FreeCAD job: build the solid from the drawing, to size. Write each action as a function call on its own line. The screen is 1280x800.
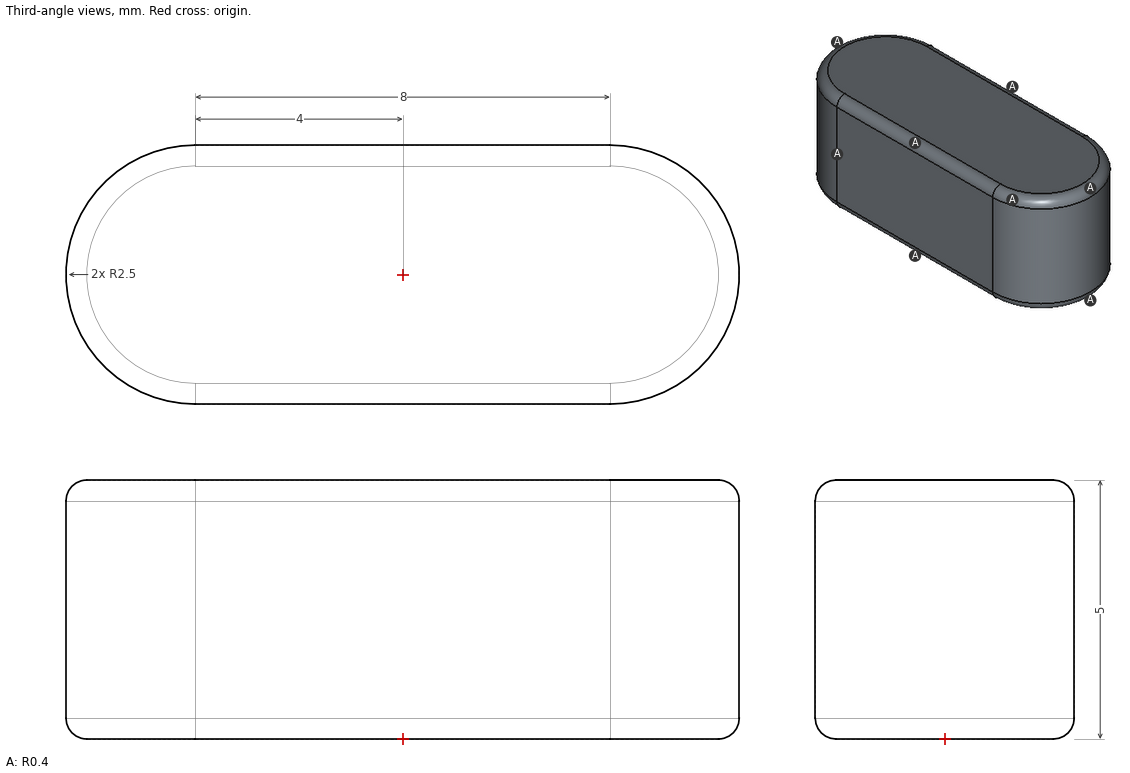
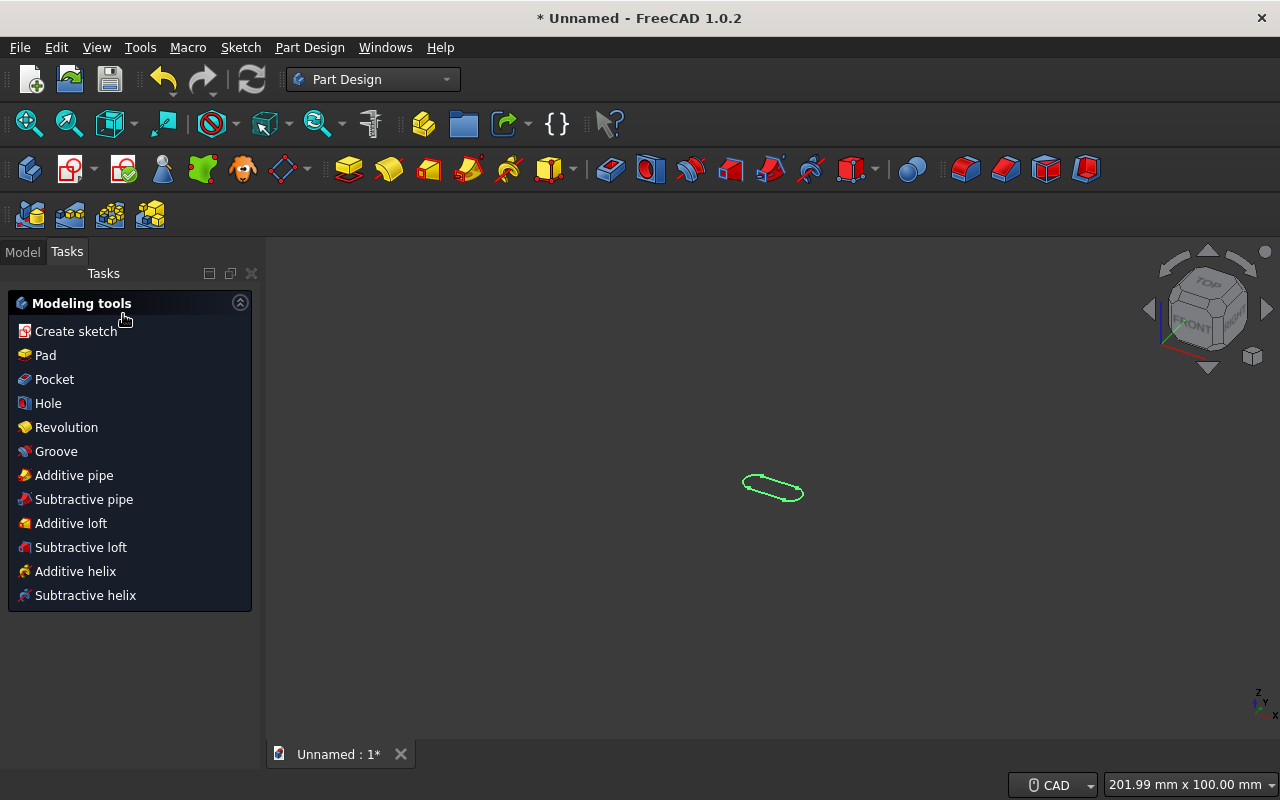
click(350, 170)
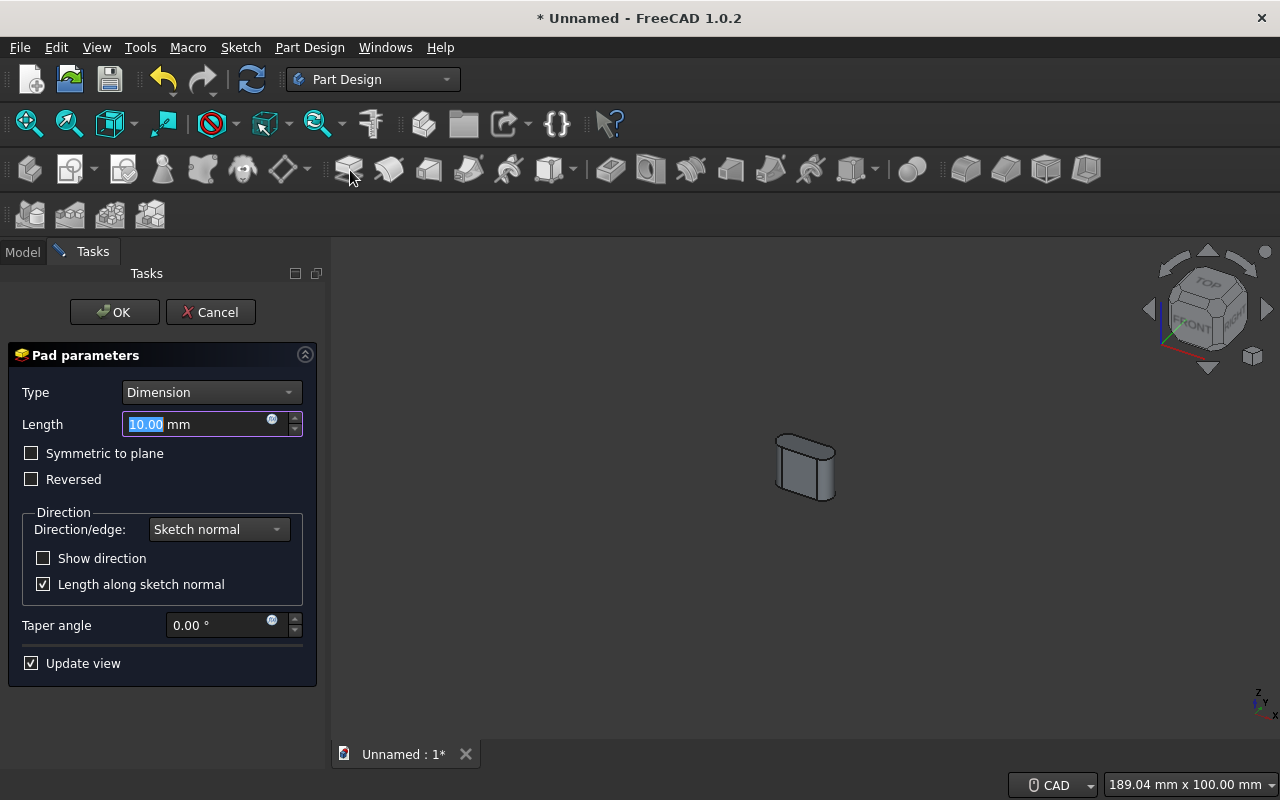
text(5)
key(Tab)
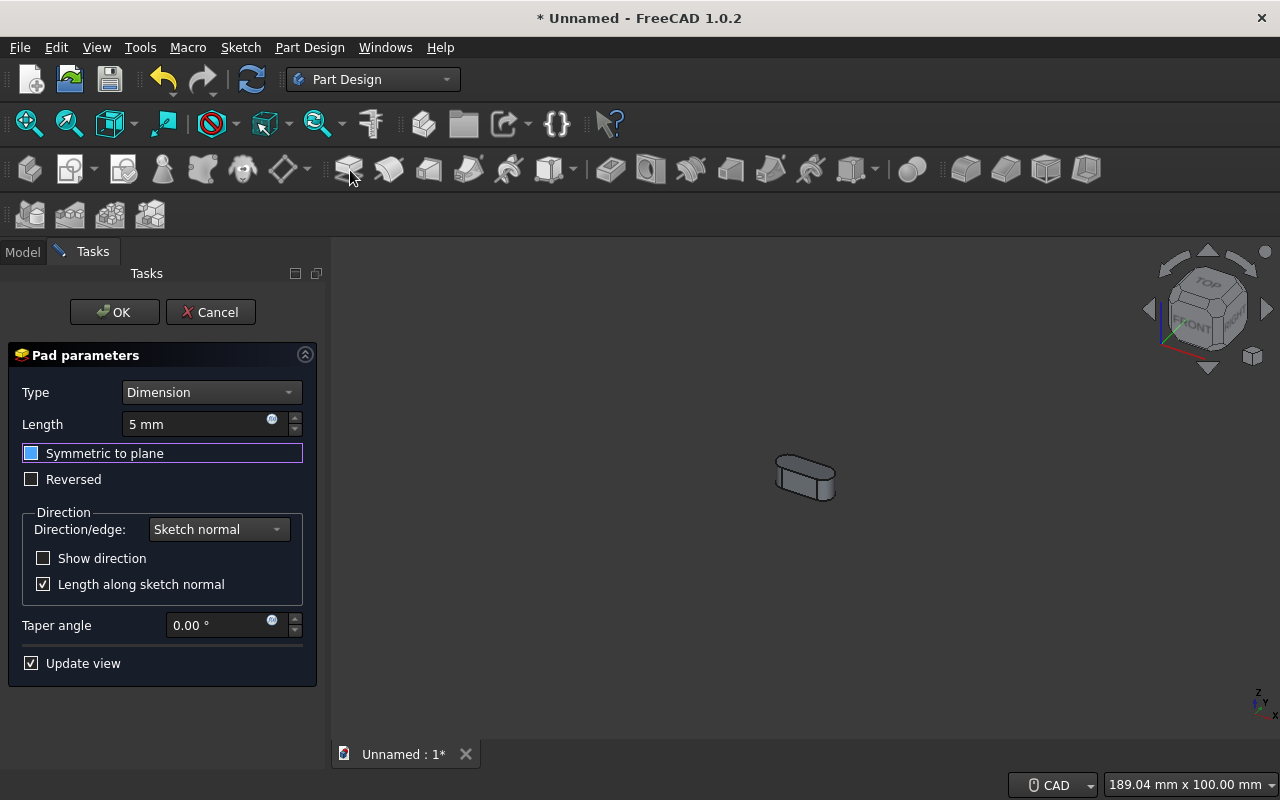
click(115, 312)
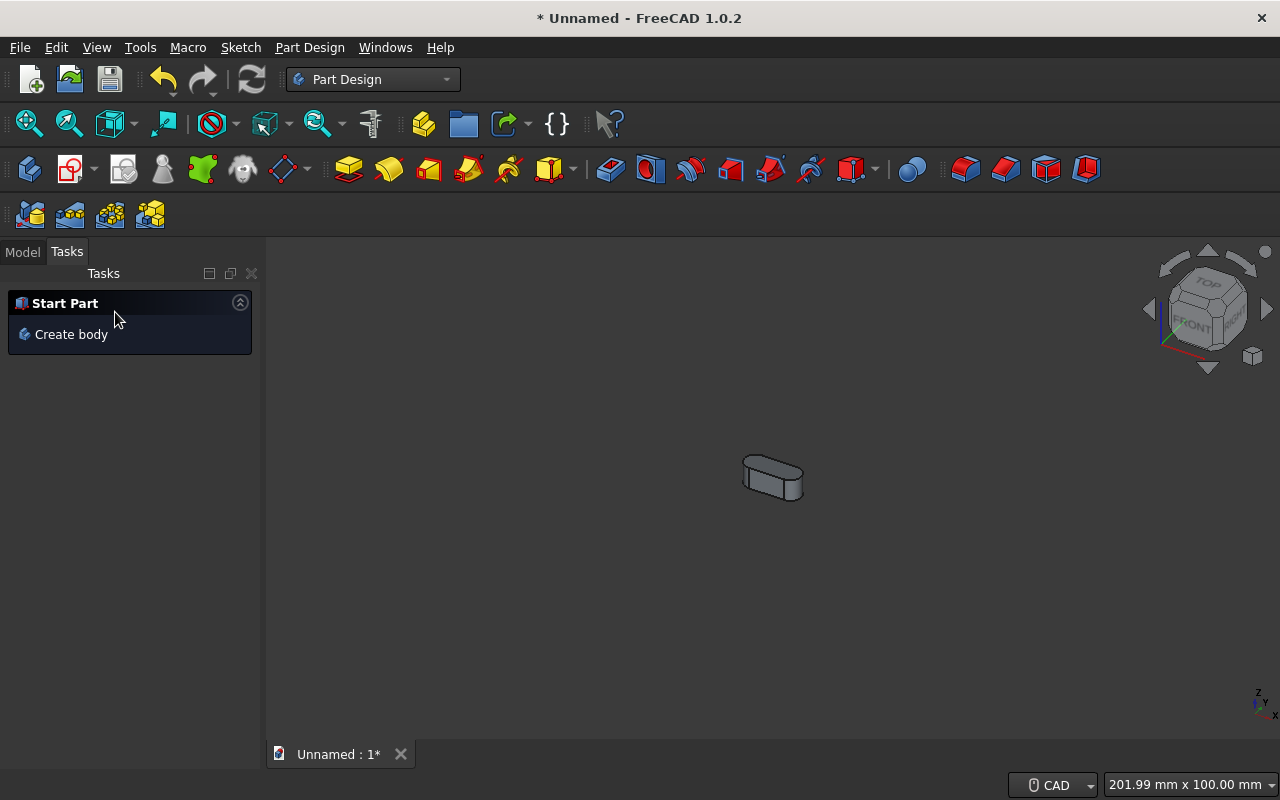
click(30, 124)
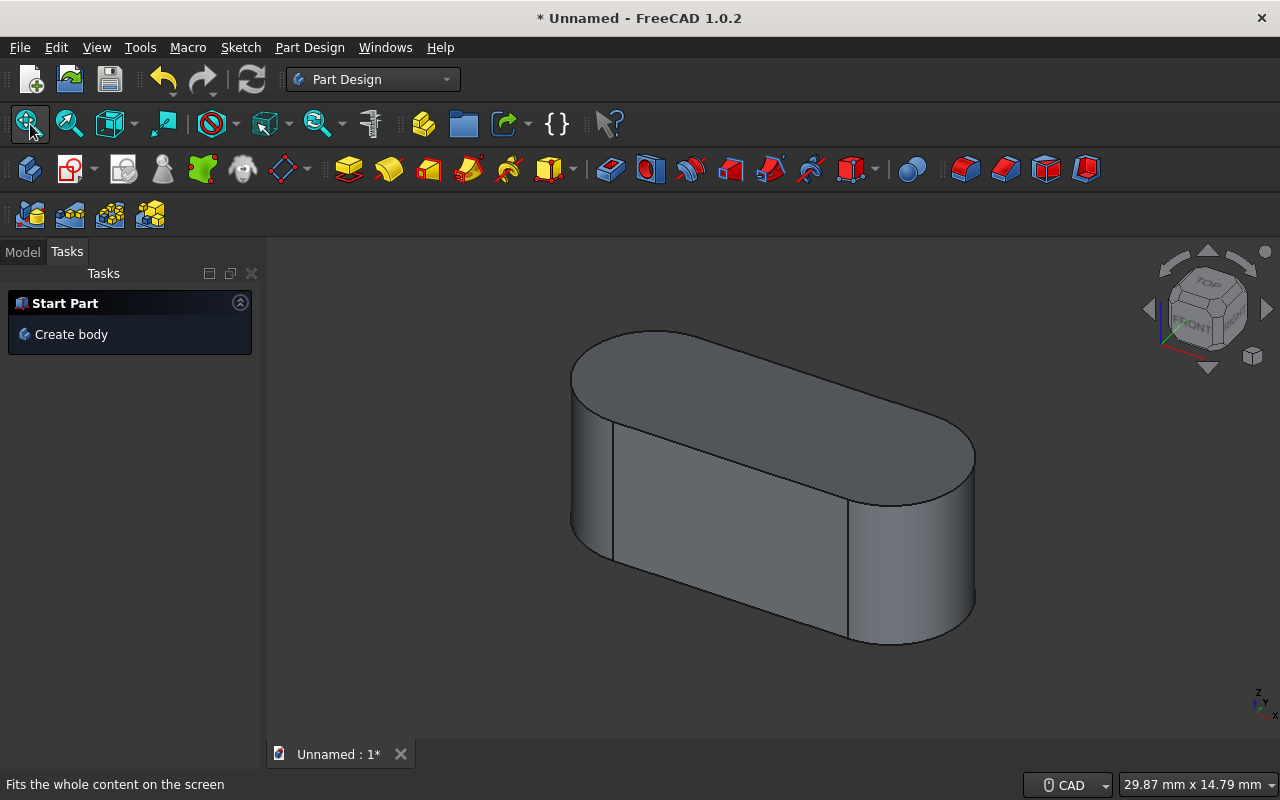
click(882, 454)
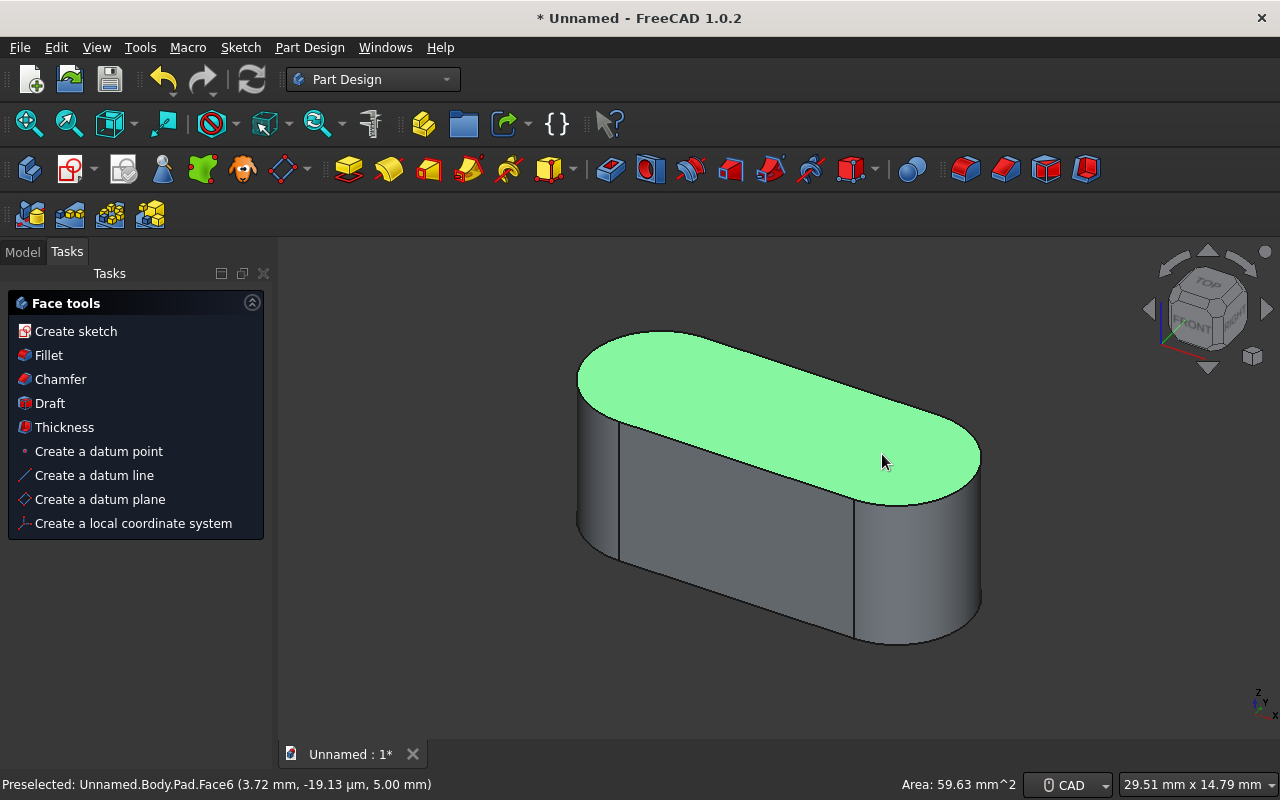
key(0)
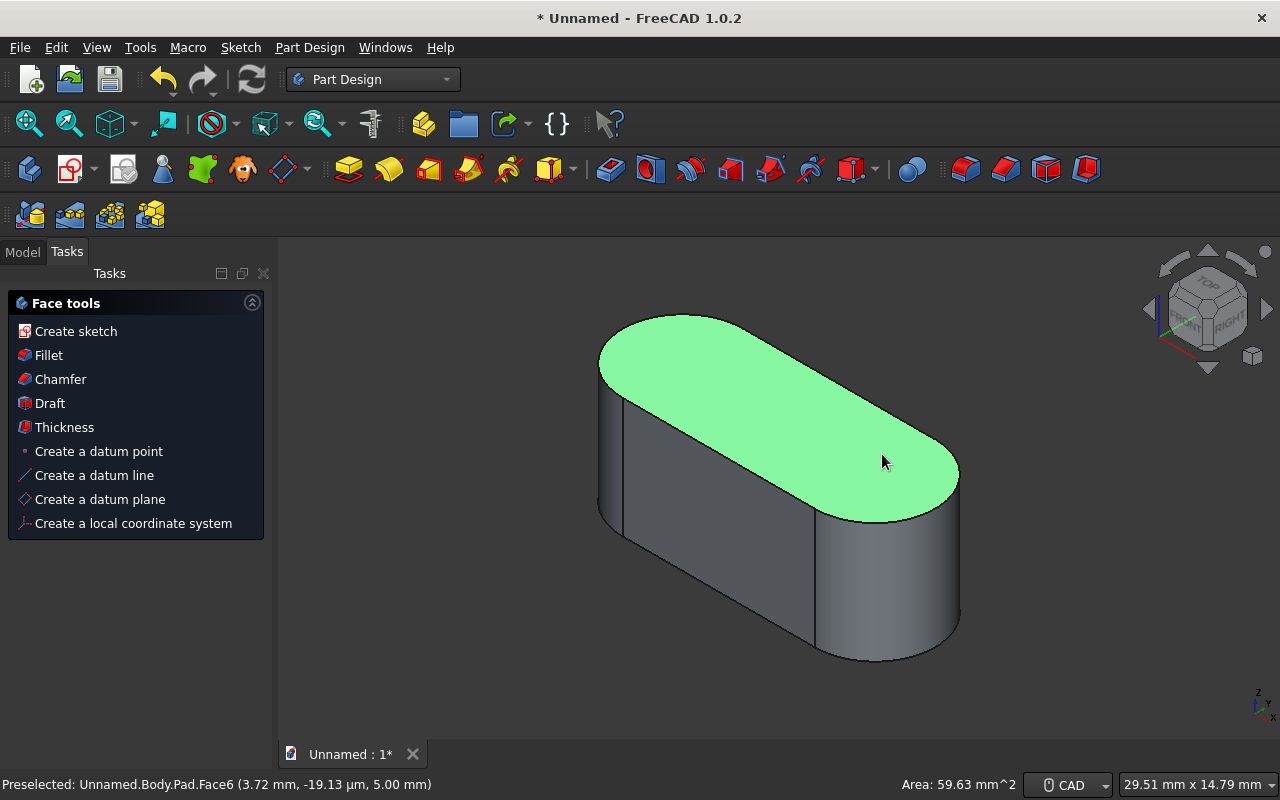
key(2)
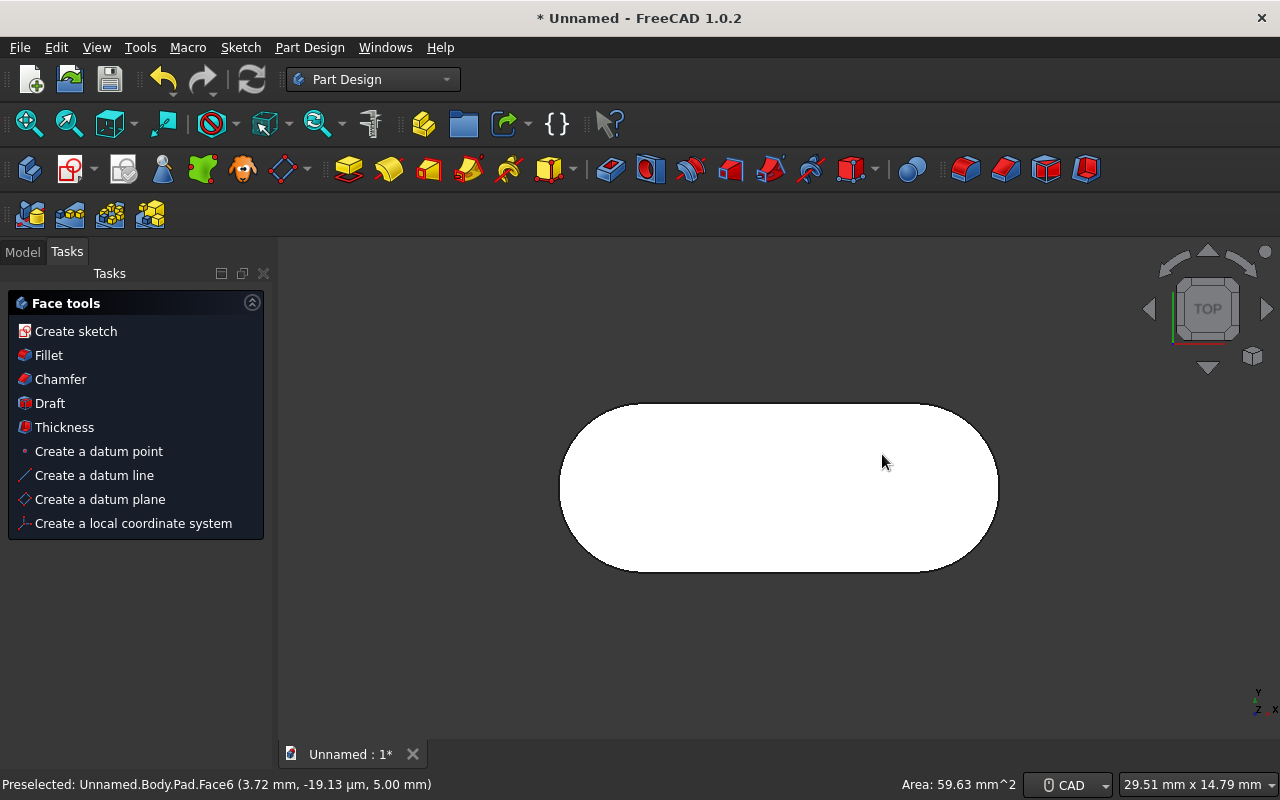
click(30, 124)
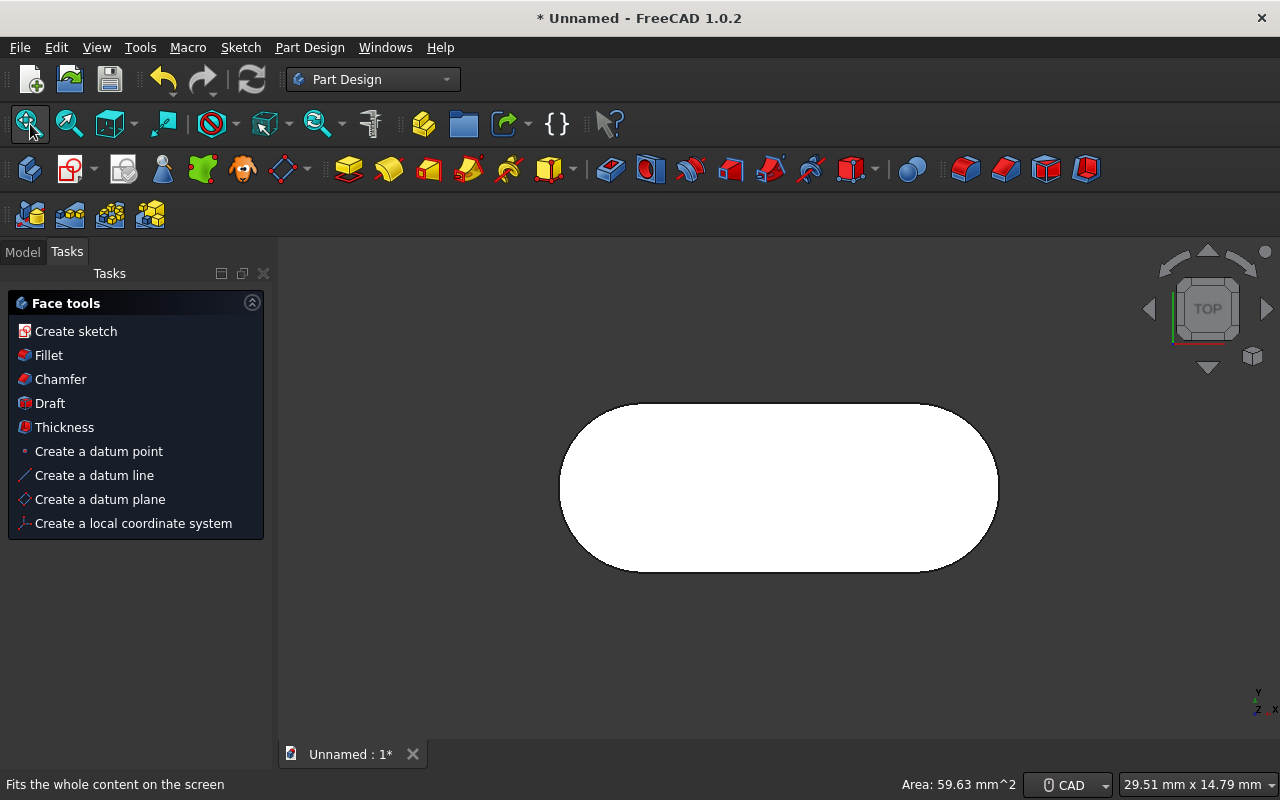
key(1)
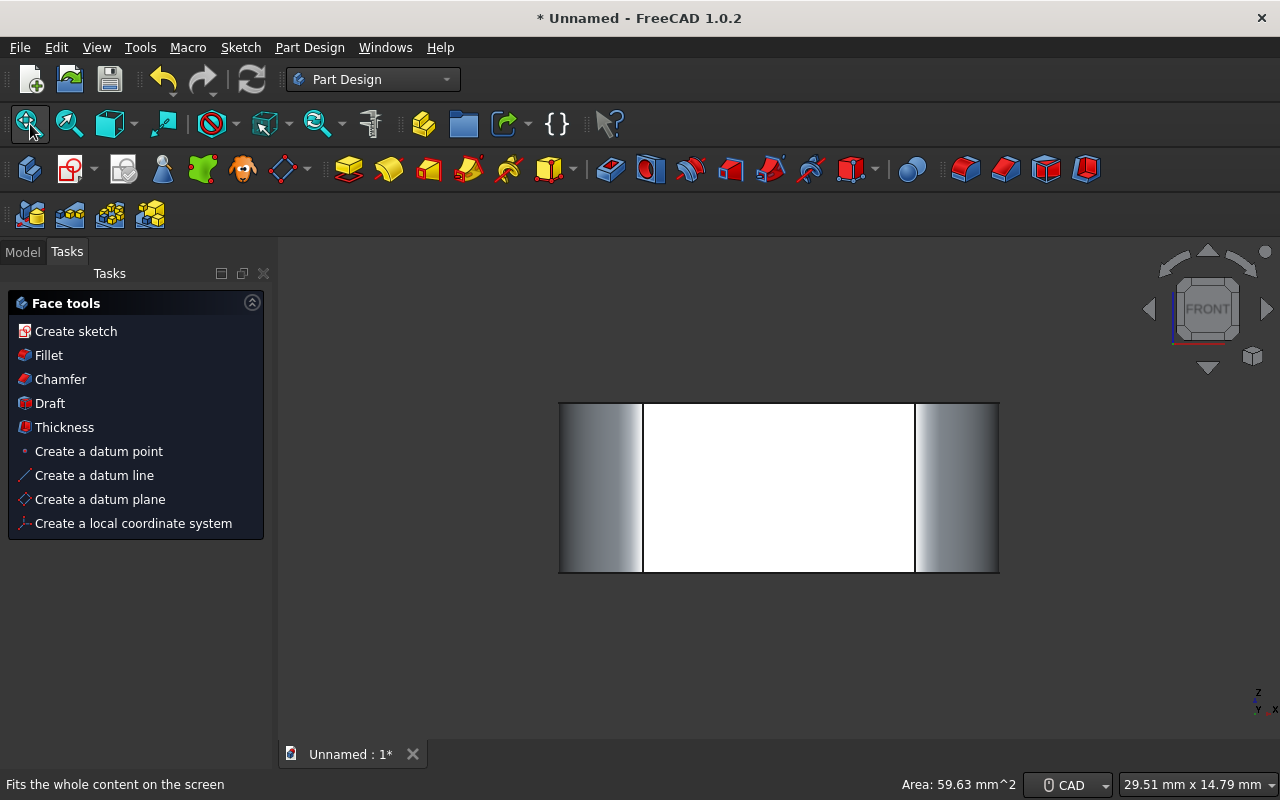
click(30, 124)